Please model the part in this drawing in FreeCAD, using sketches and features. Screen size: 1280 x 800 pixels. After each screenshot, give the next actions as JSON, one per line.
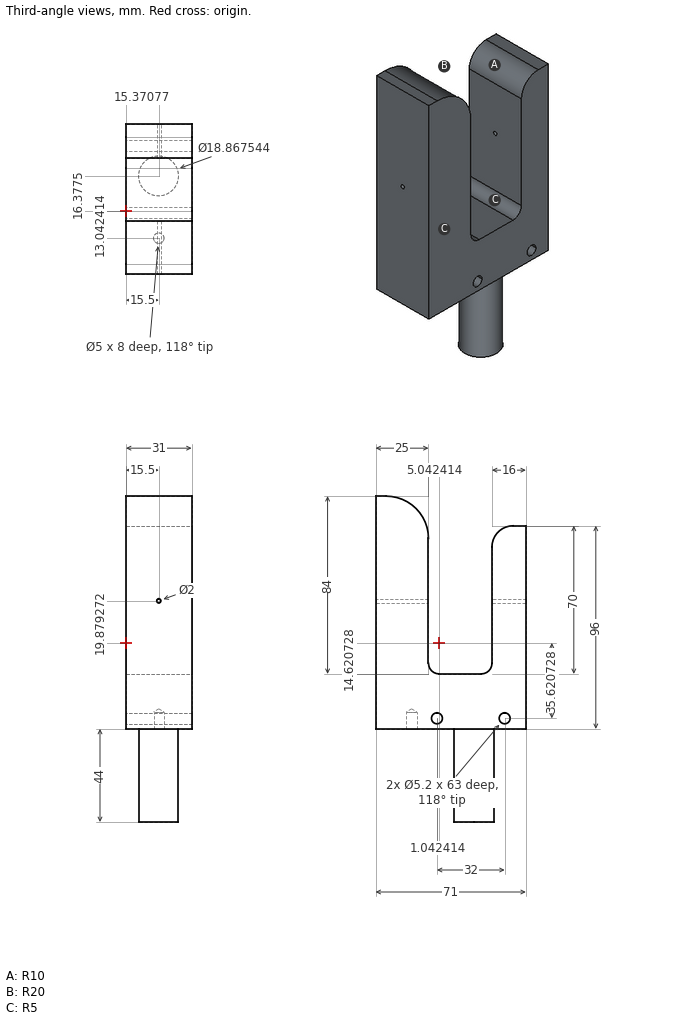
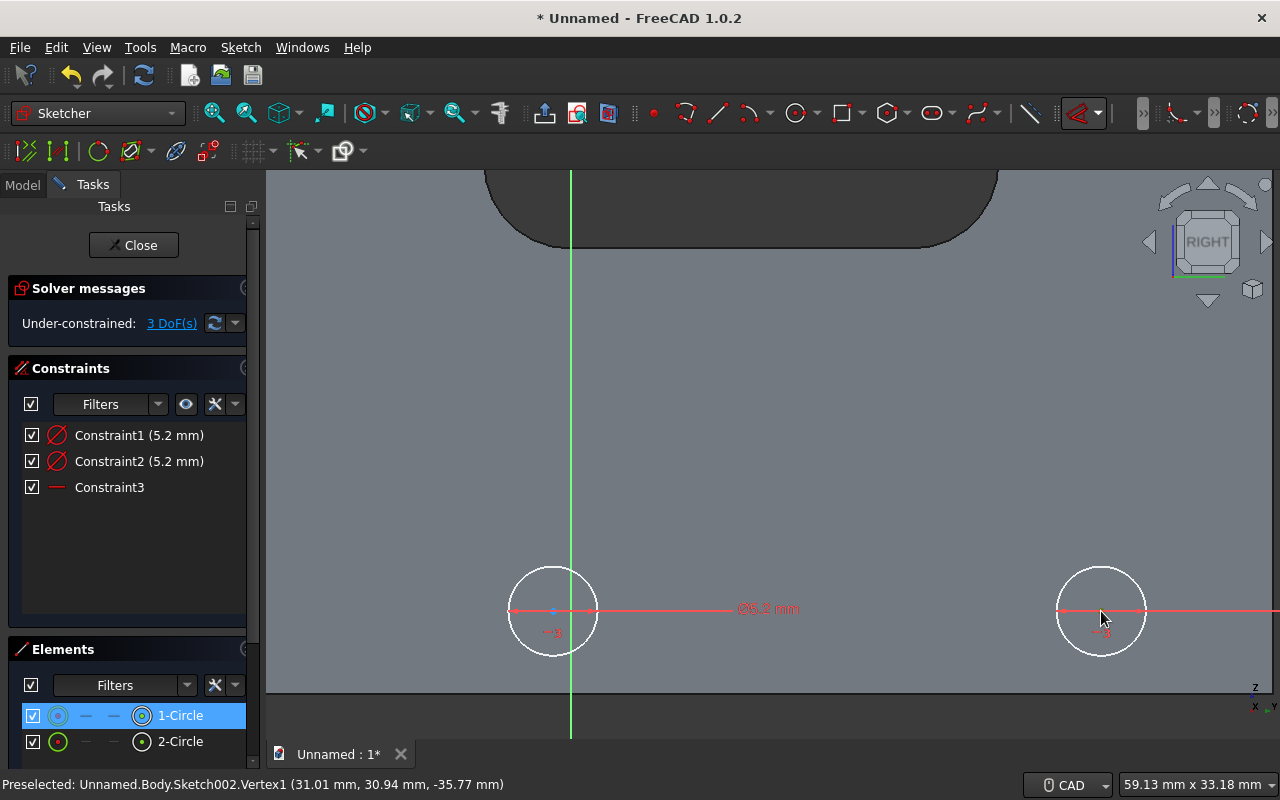
{"action": "left_click", "coordinate": [553, 611]}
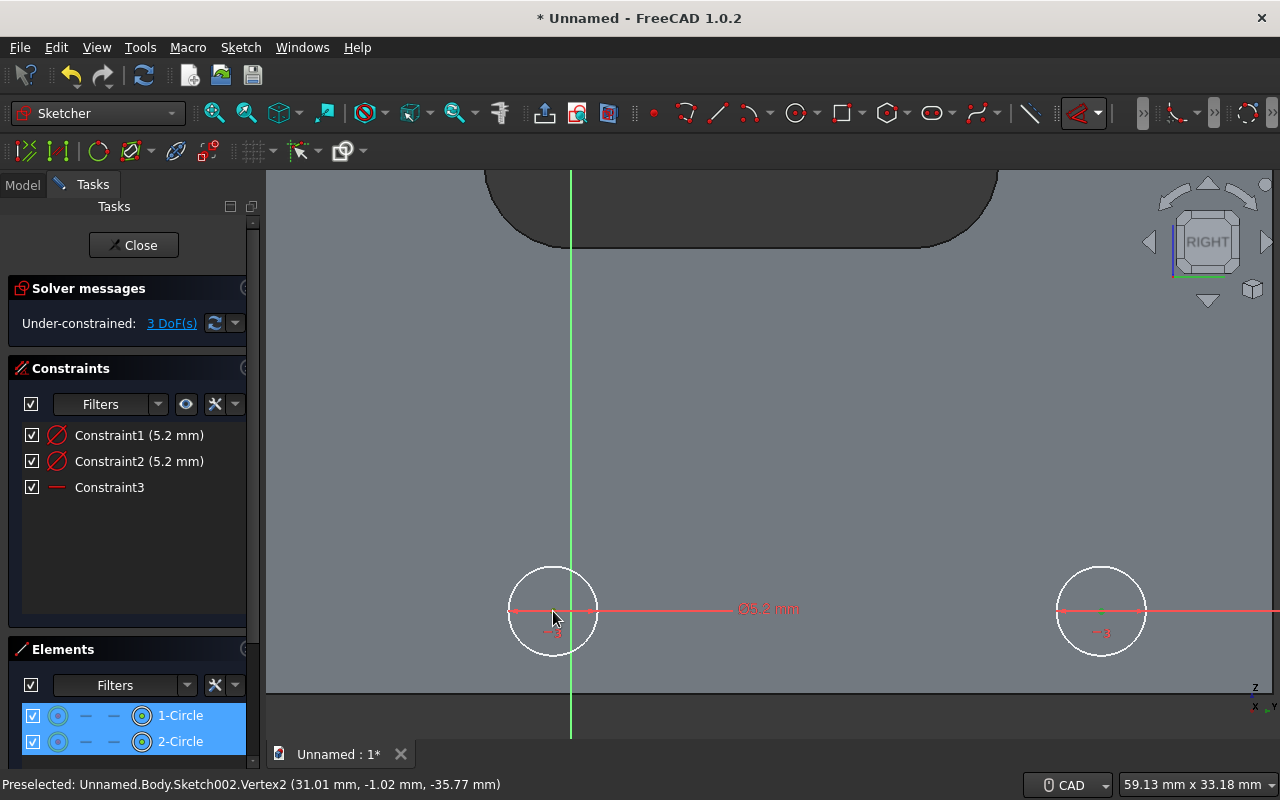
{"action": "key", "text": "l"}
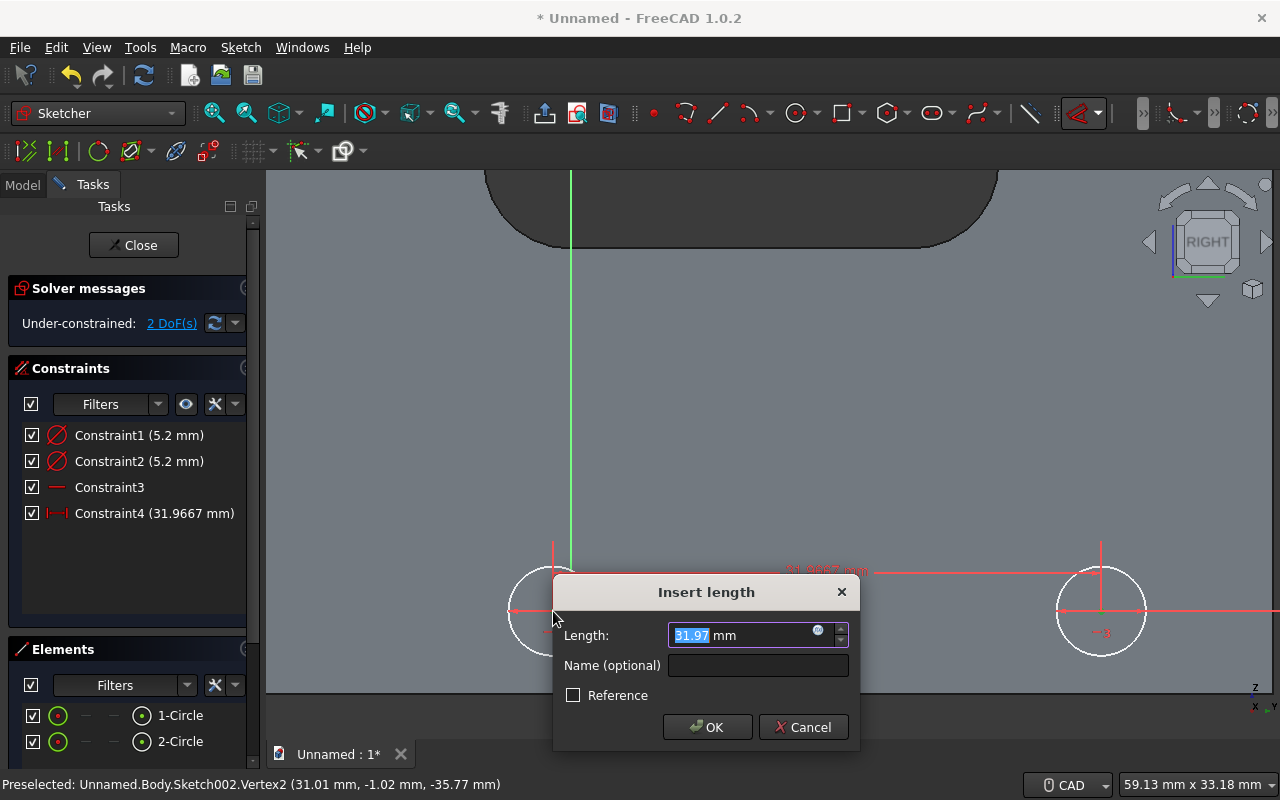
{"action": "type", "text": "32"}
{"action": "key", "text": "Return"}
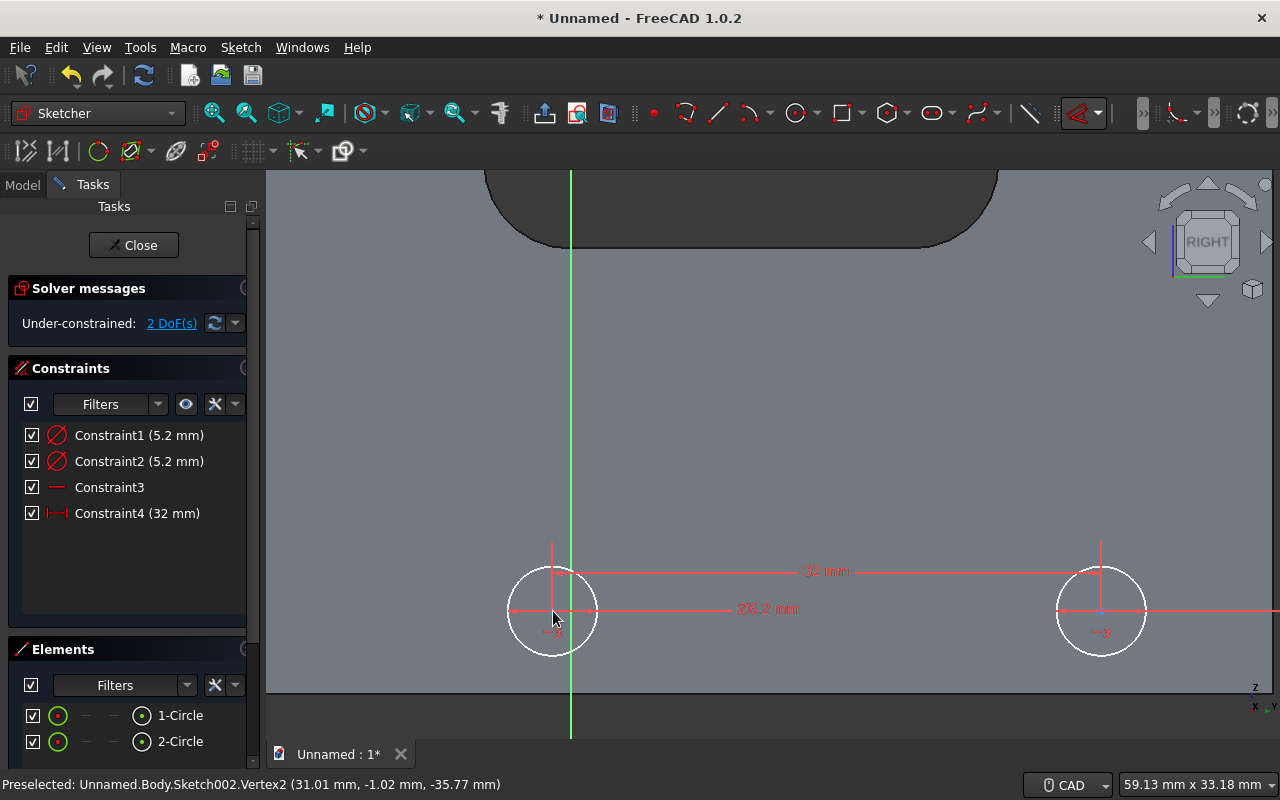
{"action": "scroll", "coordinate": [552, 611], "scroll_direction": "up", "scroll_amount": 4}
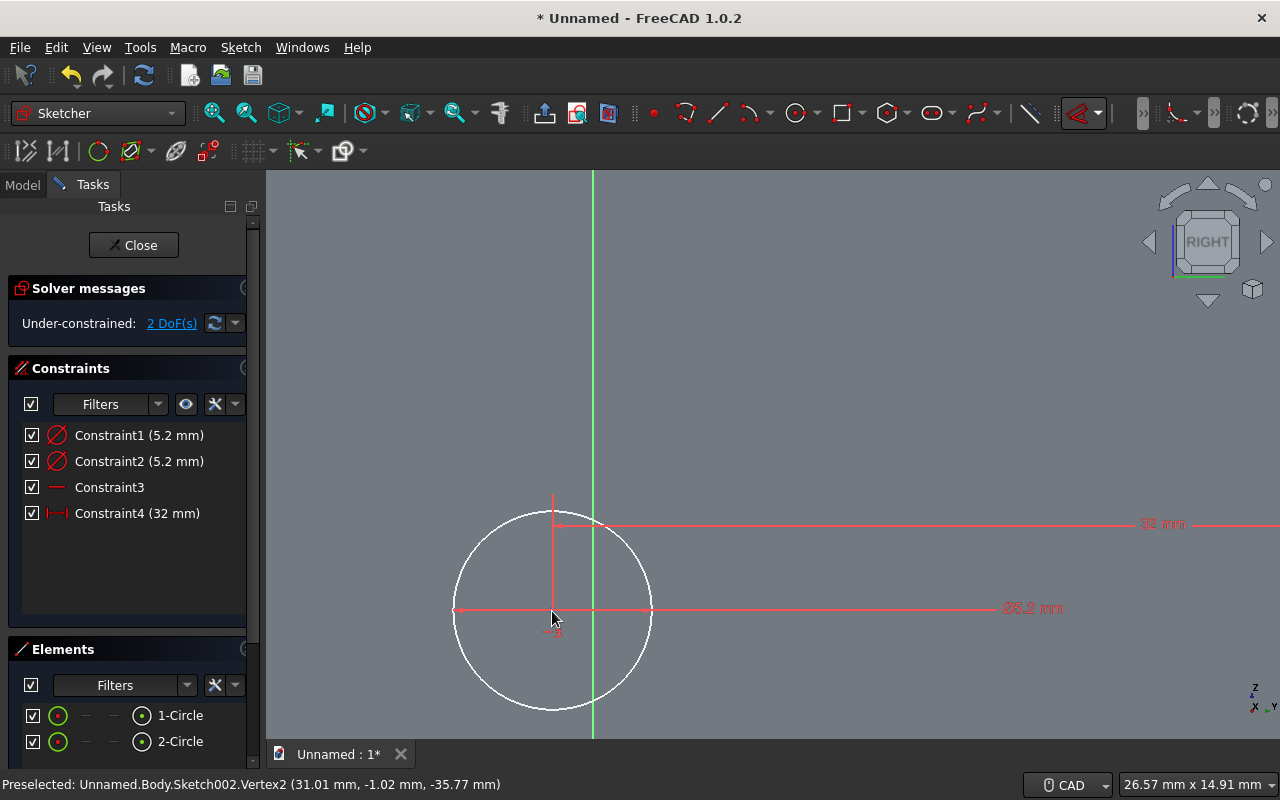
{"action": "left_click", "coordinate": [553, 610]}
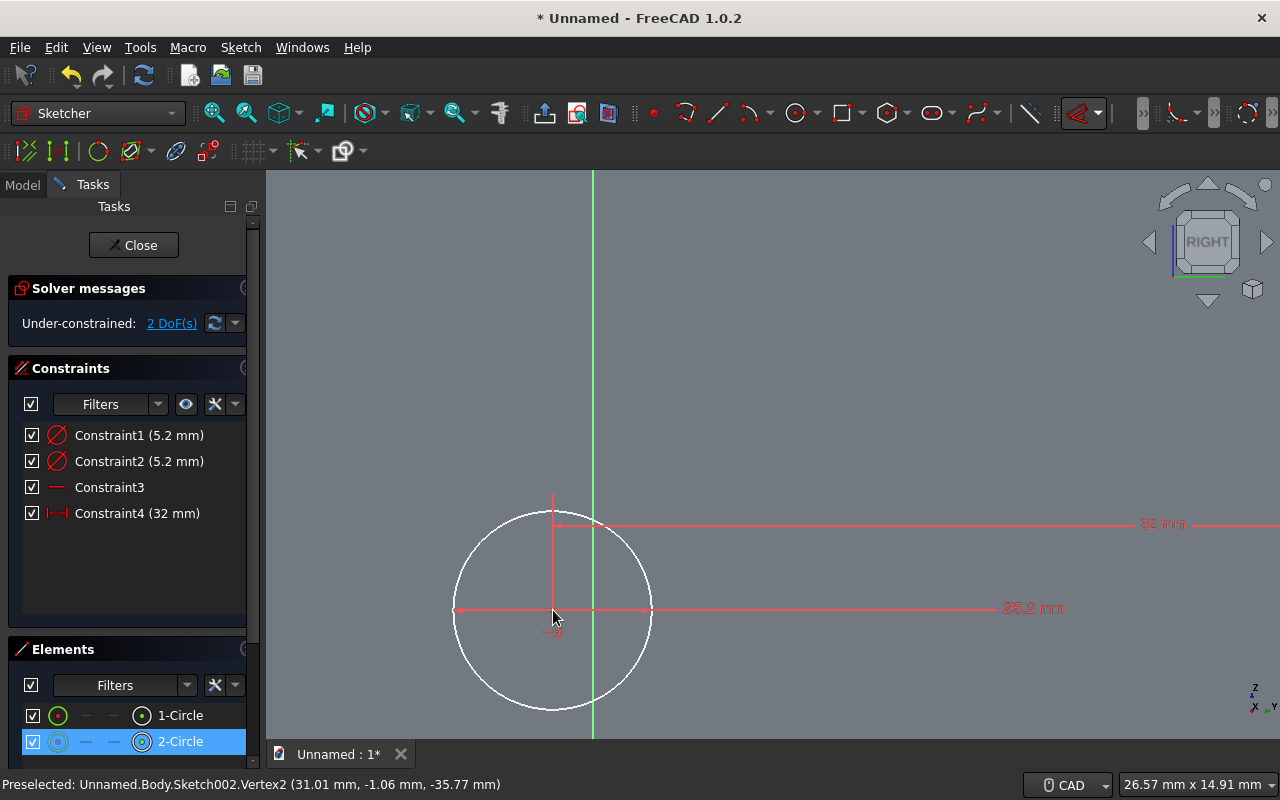
{"action": "left_click", "coordinate": [1100, 114]}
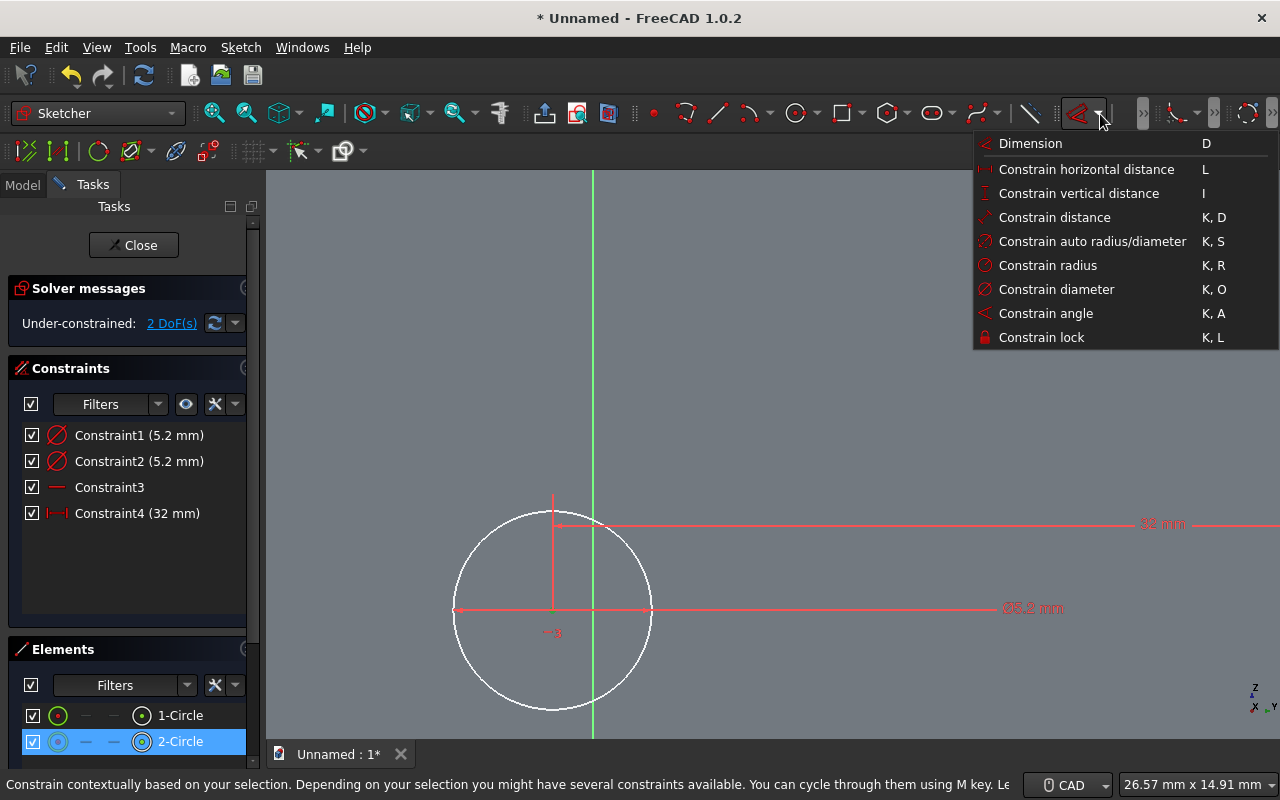
{"action": "left_click", "coordinate": [1126, 169]}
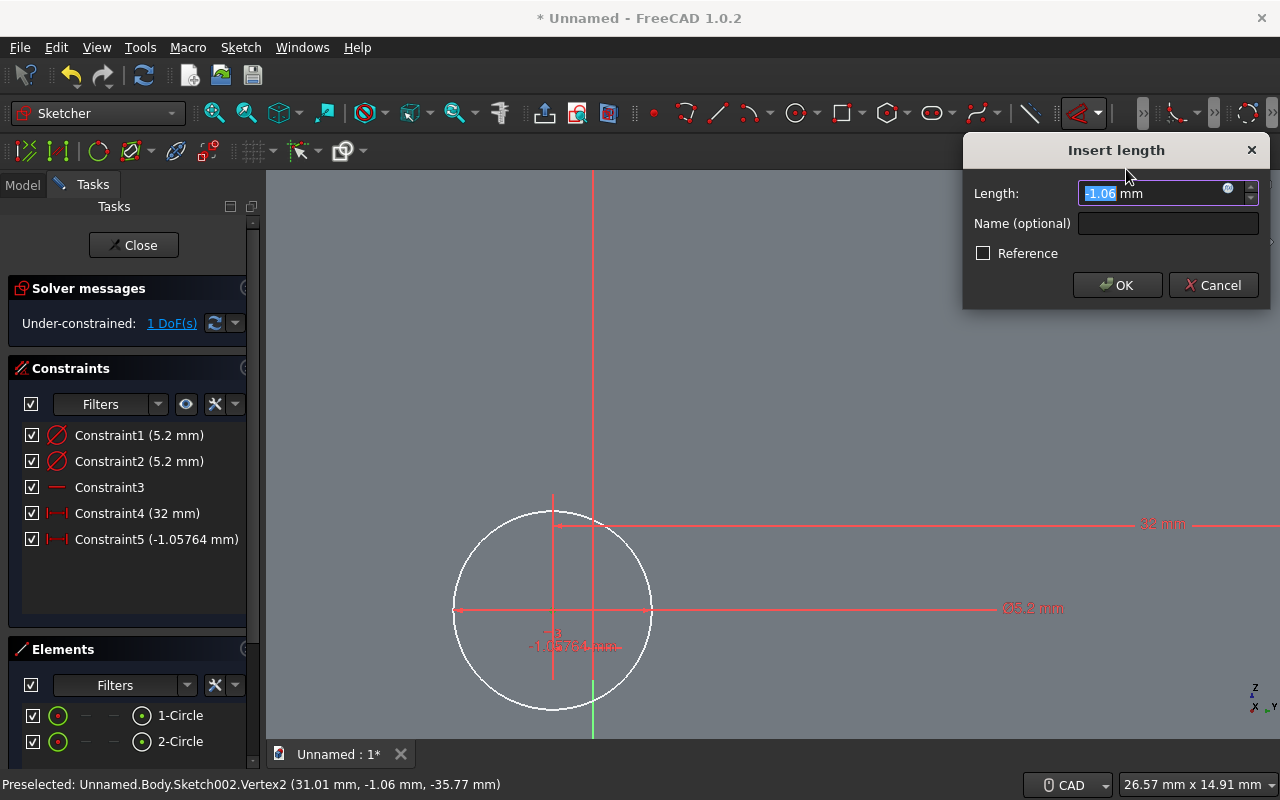
{"action": "type", "text": "-1.042414"}
{"action": "key", "text": "Return"}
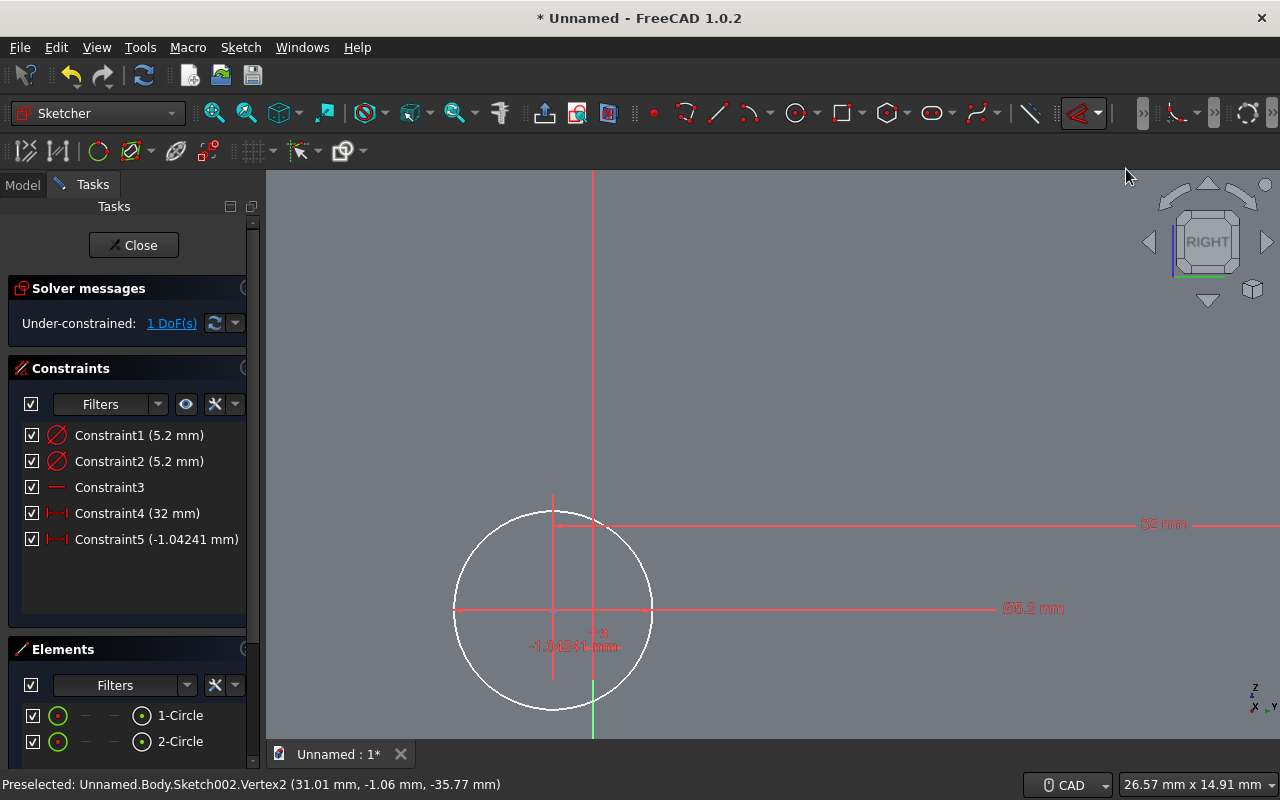
{"action": "scroll", "coordinate": [554, 612], "scroll_direction": "down", "scroll_amount": 7}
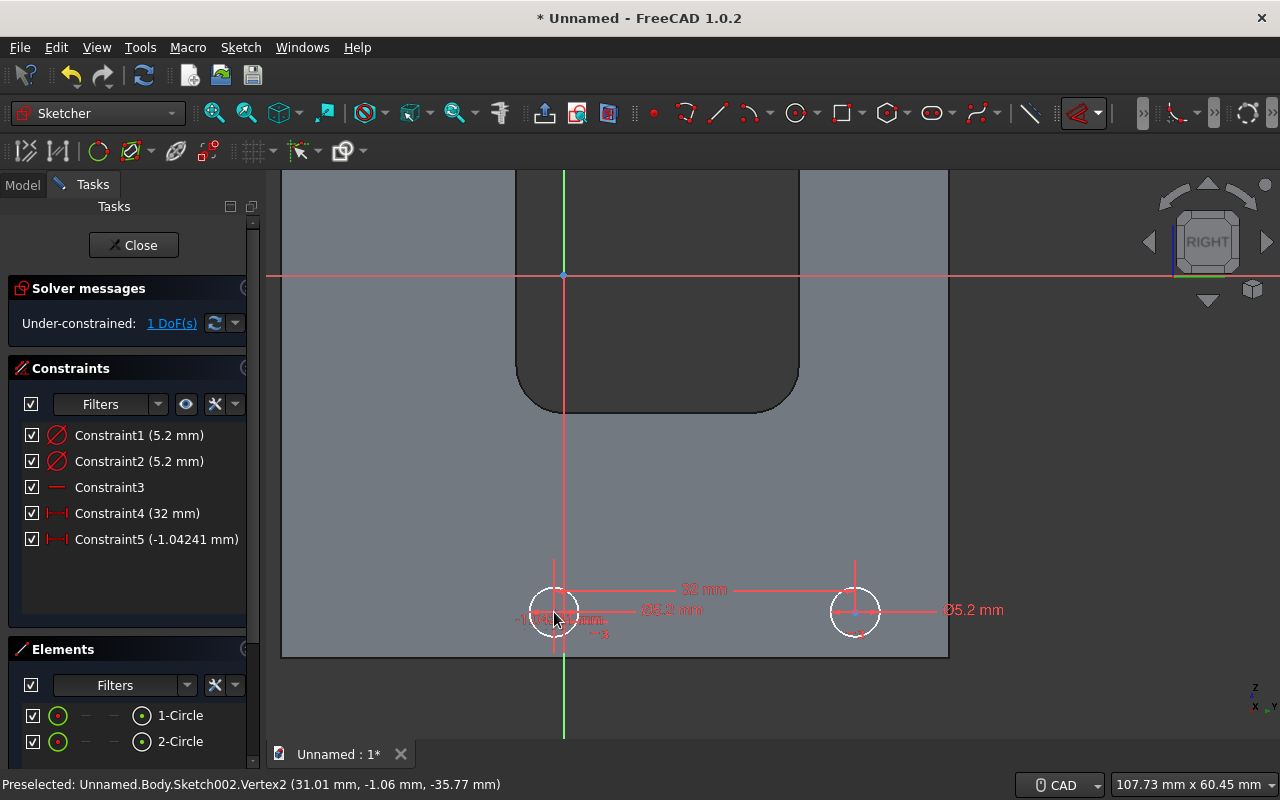
{"action": "left_click", "coordinate": [855, 612]}